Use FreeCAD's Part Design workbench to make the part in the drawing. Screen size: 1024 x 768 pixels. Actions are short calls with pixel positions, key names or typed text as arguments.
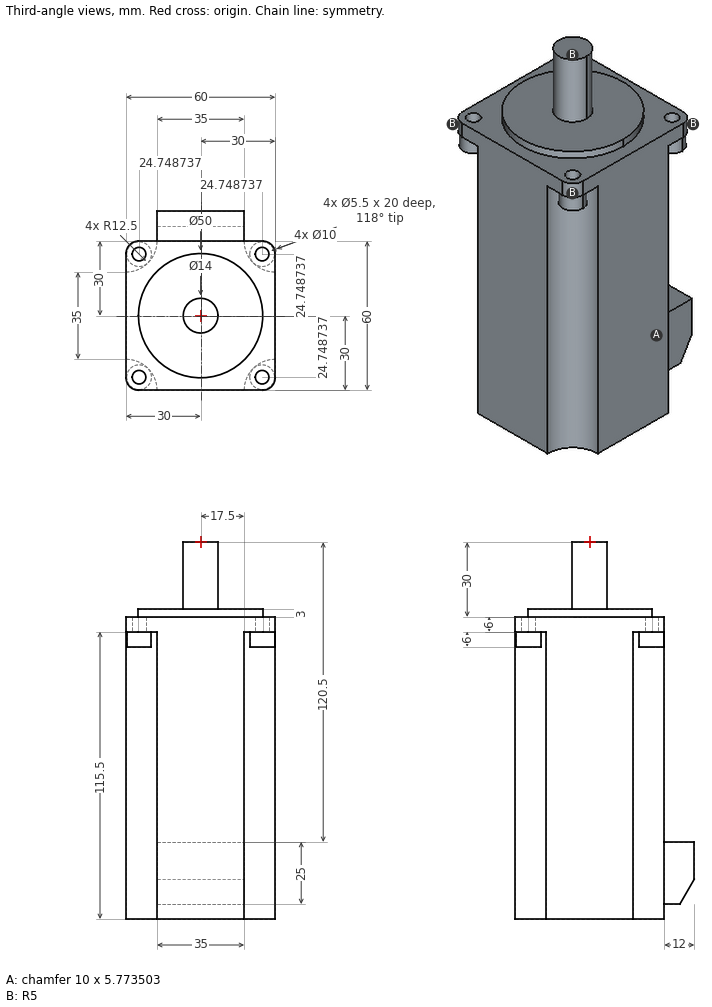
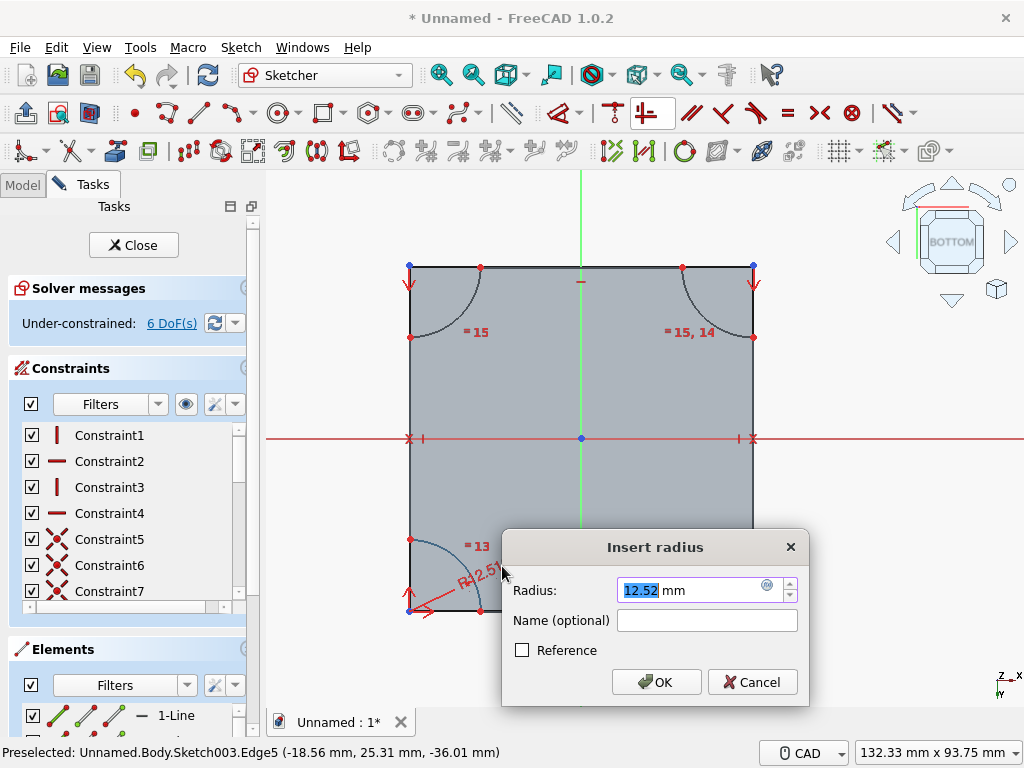
text(12.5)
key(Return)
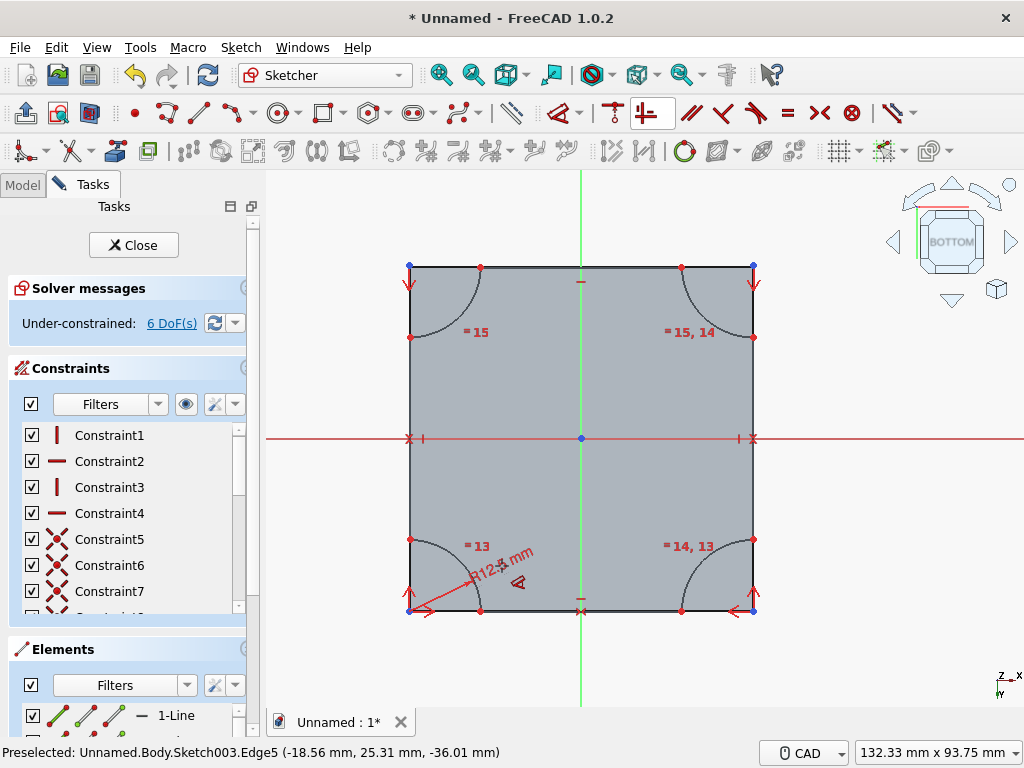
click(410, 398)
click(376, 392)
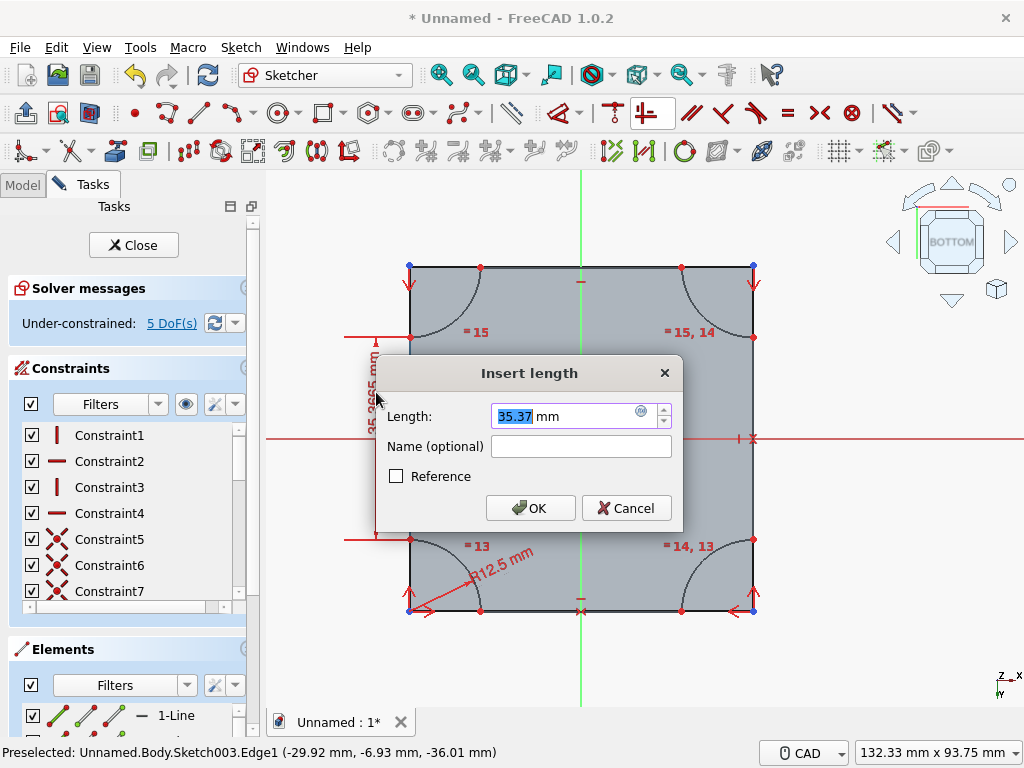
text(35)
key(Return)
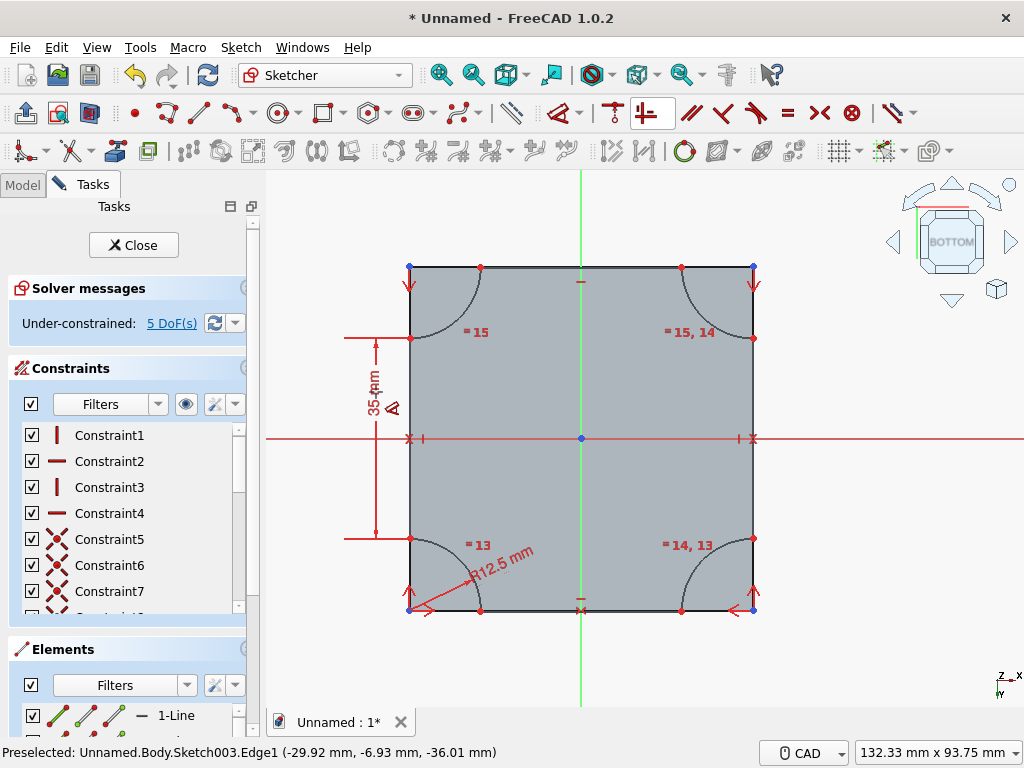
click(541, 612)
click(535, 646)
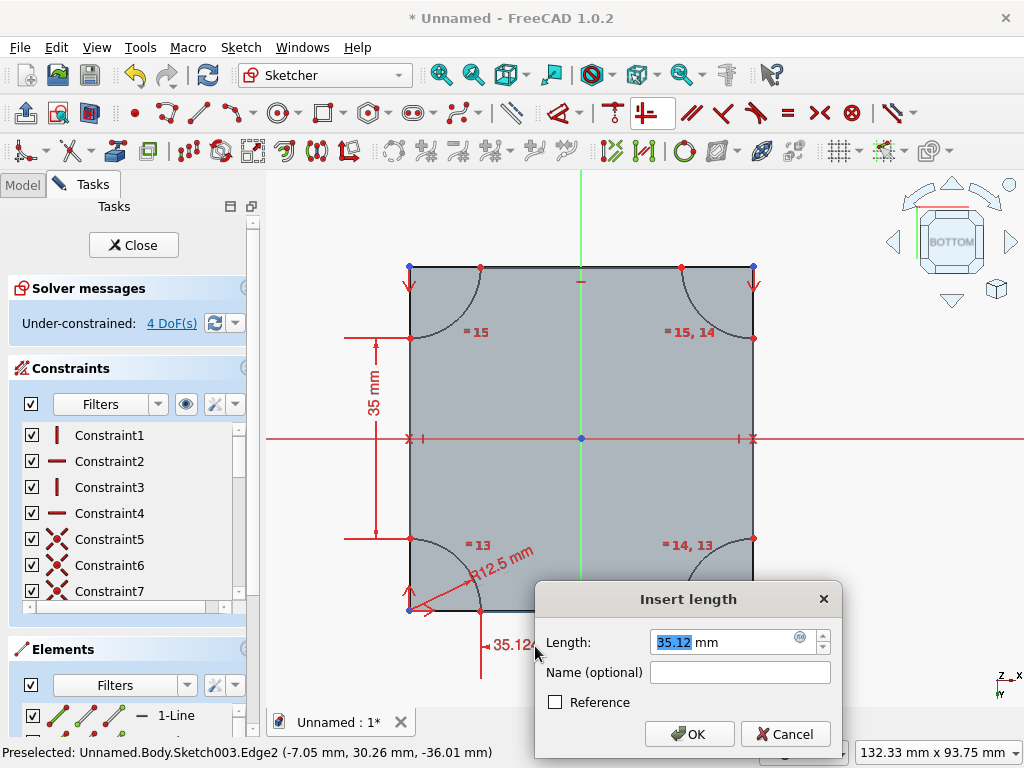
text(35)
key(Return)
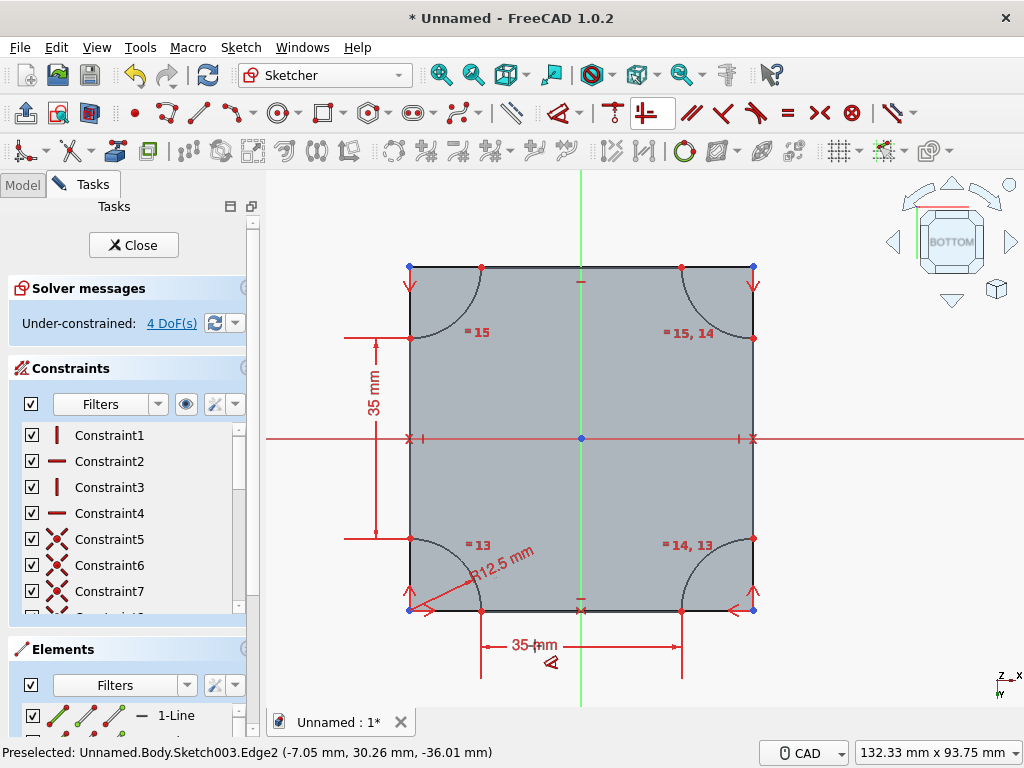
click(410, 338)
click(496, 304)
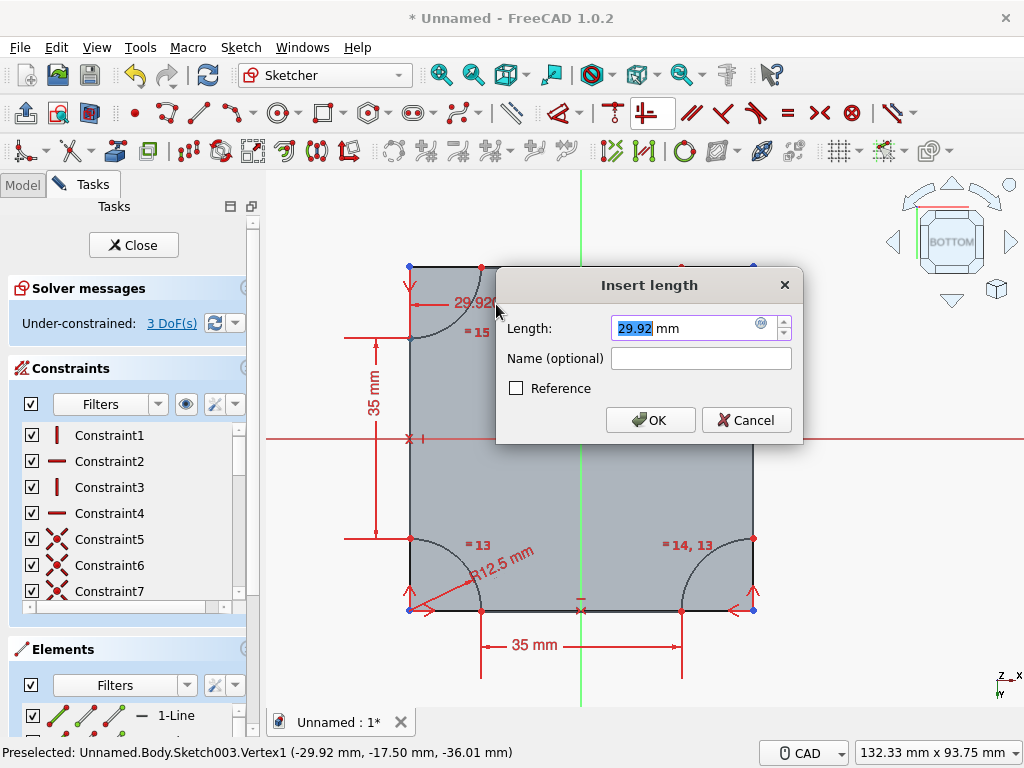
text(30)
key(Return)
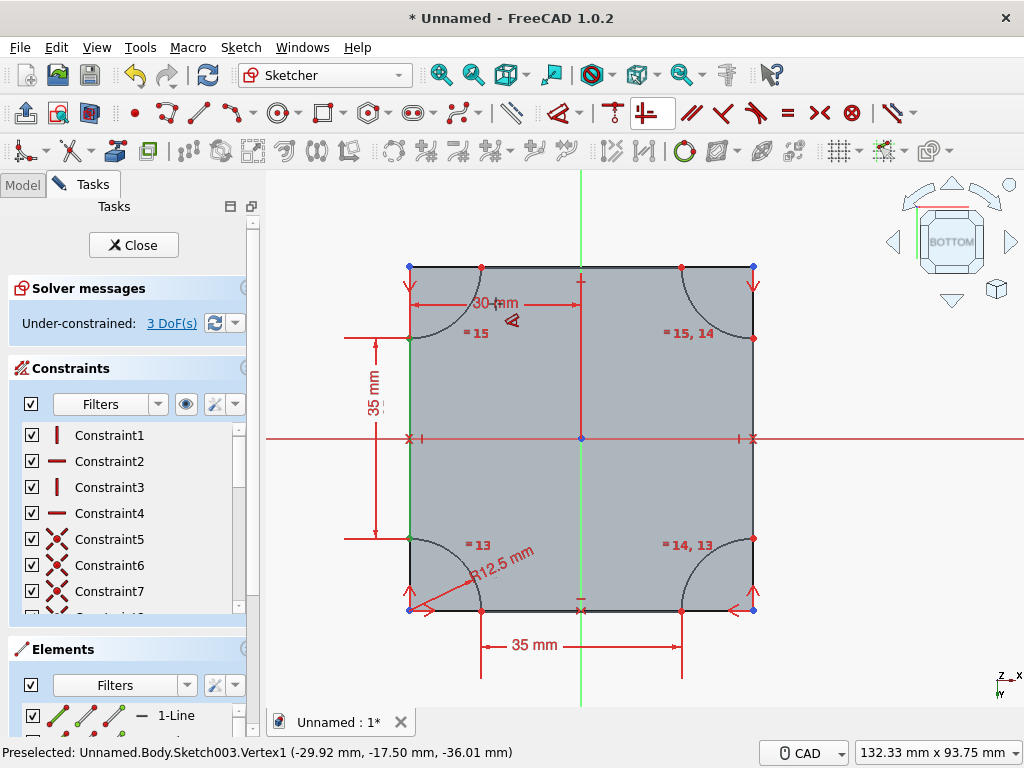
click(481, 612)
click(447, 525)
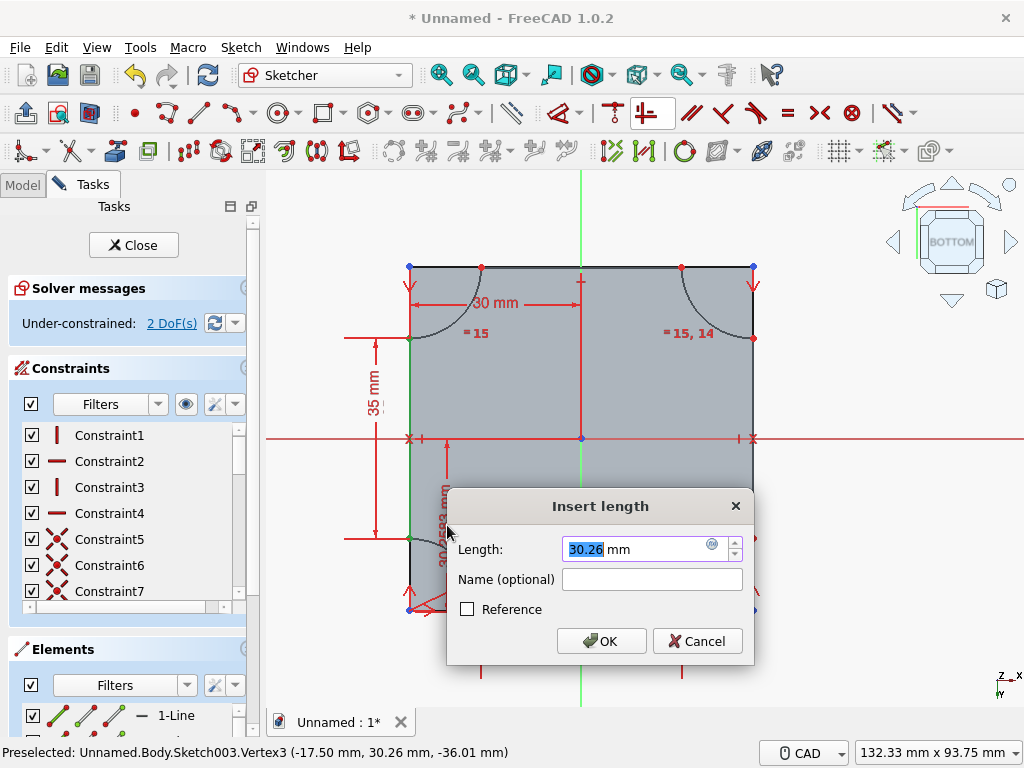
text(30)
key(Return)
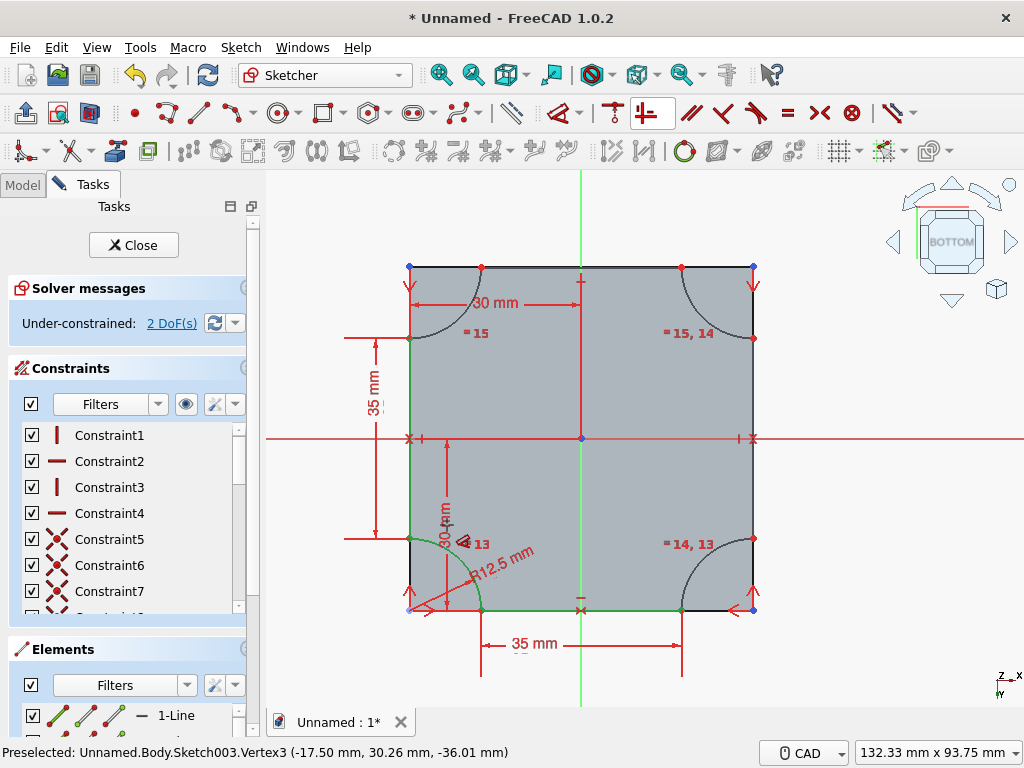
click(753, 539)
click(667, 573)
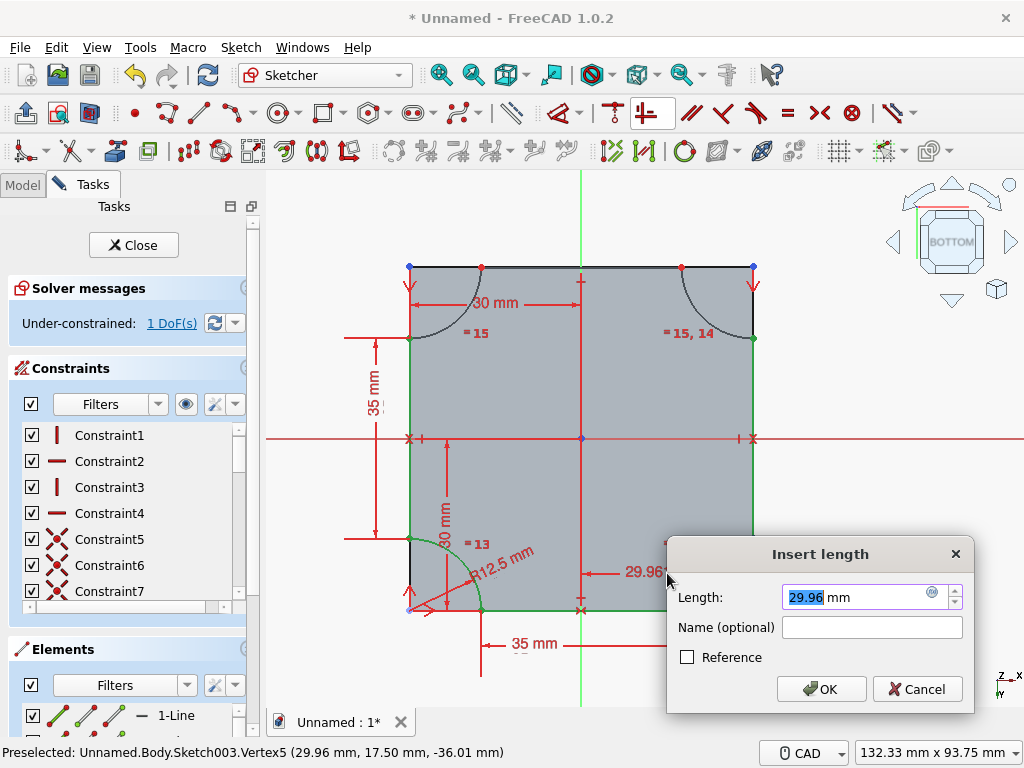
text(30)
key(Return)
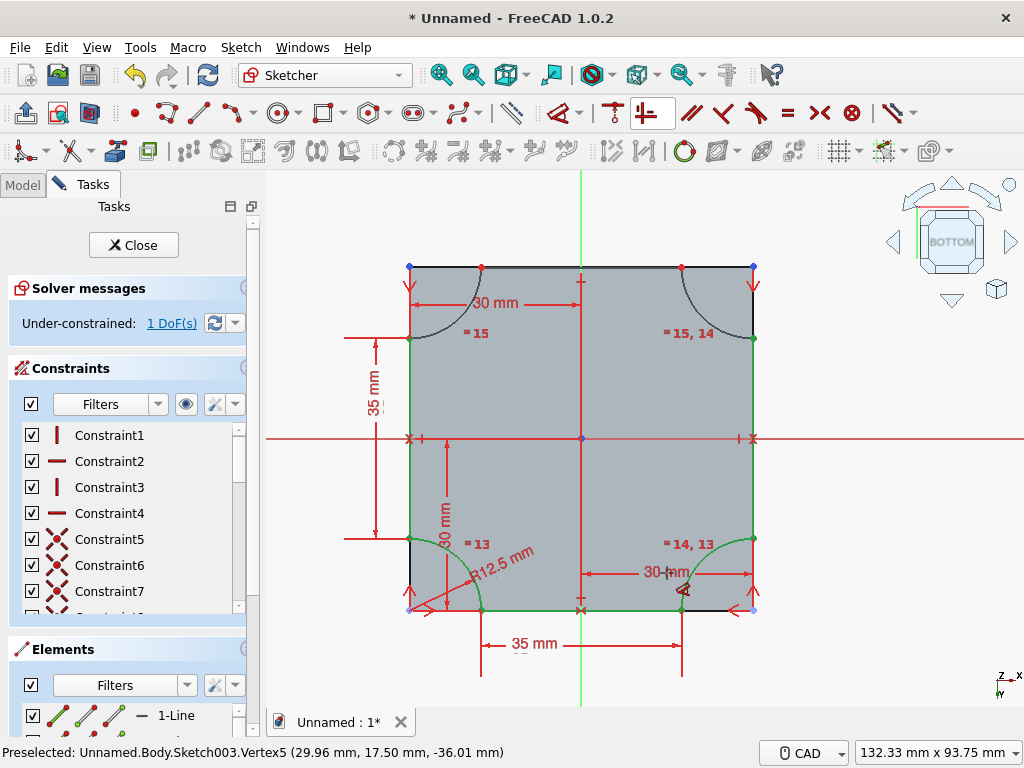
click(682, 268)
click(716, 353)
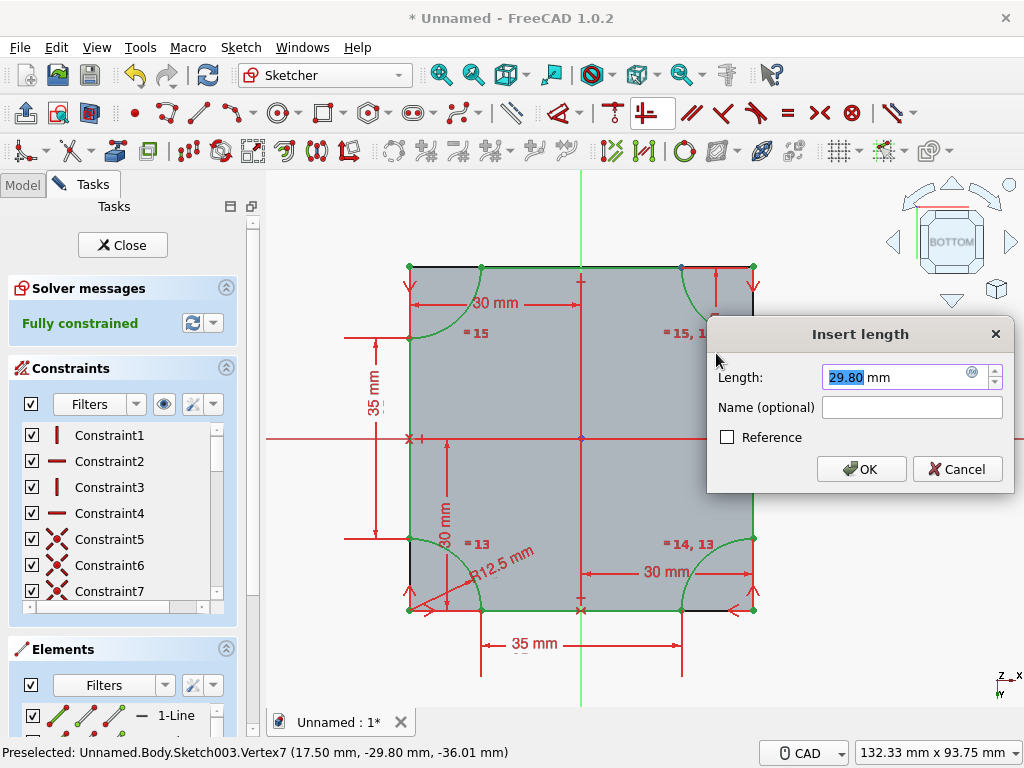
text(30)
key(Return)
key(Escape)